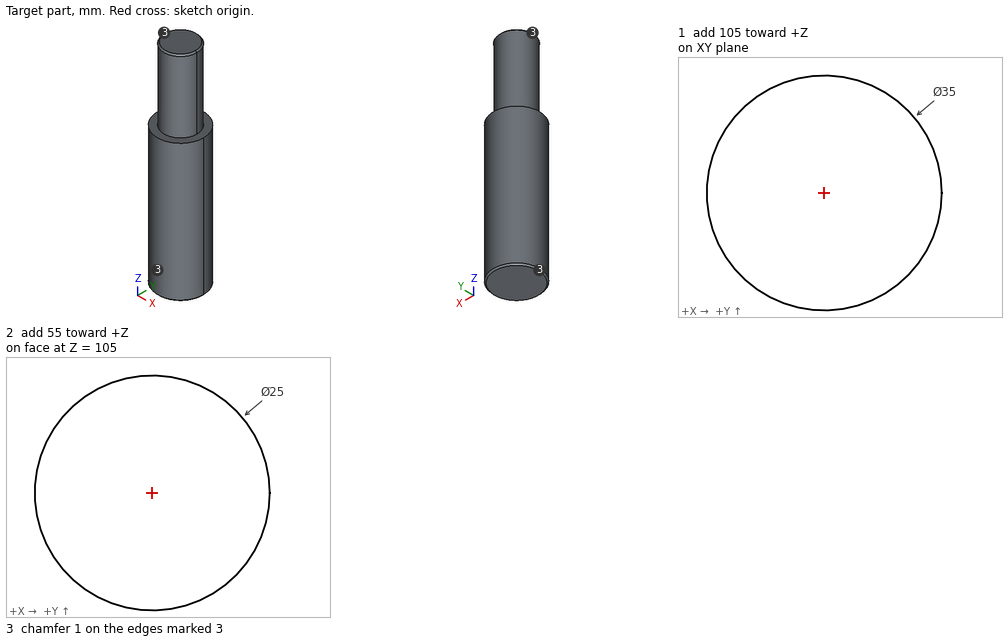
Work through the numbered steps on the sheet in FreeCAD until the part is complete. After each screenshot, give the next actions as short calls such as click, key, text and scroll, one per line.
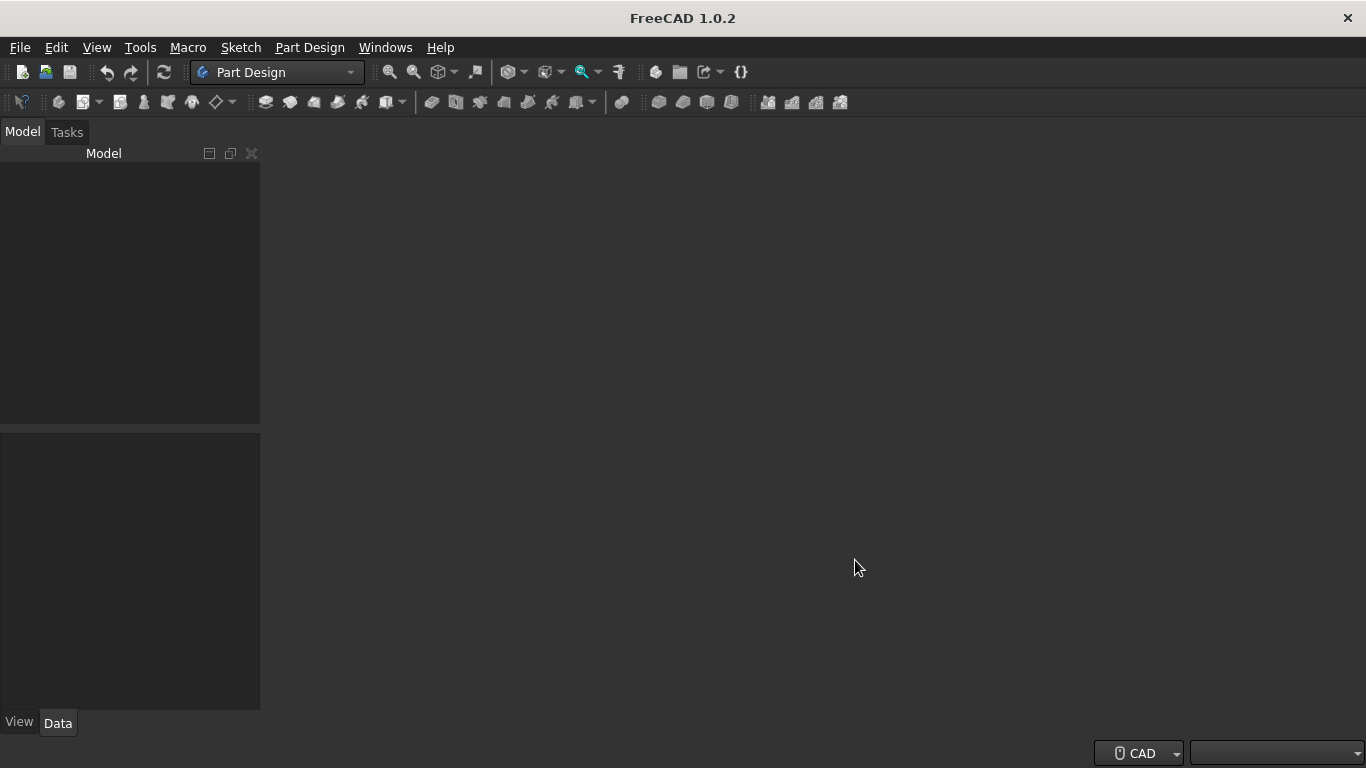
click(22, 72)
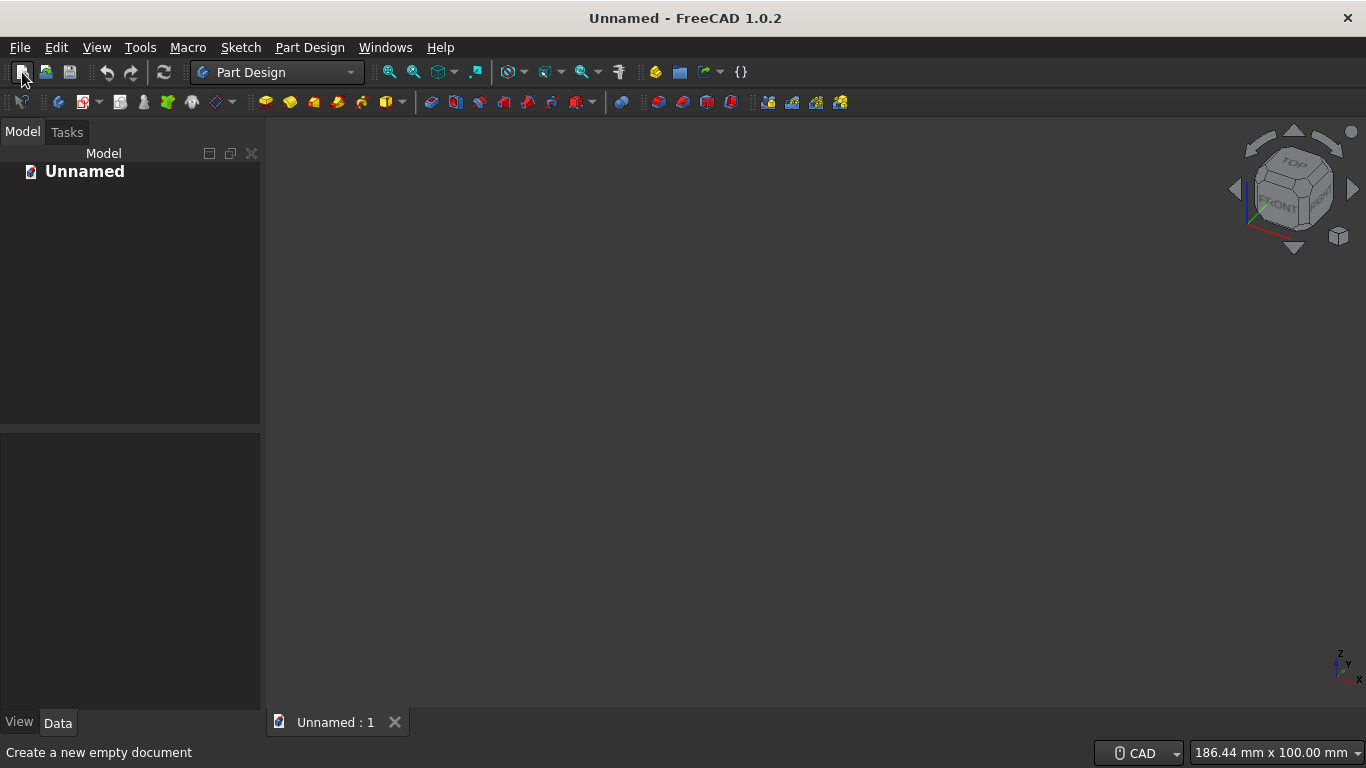
click(84, 102)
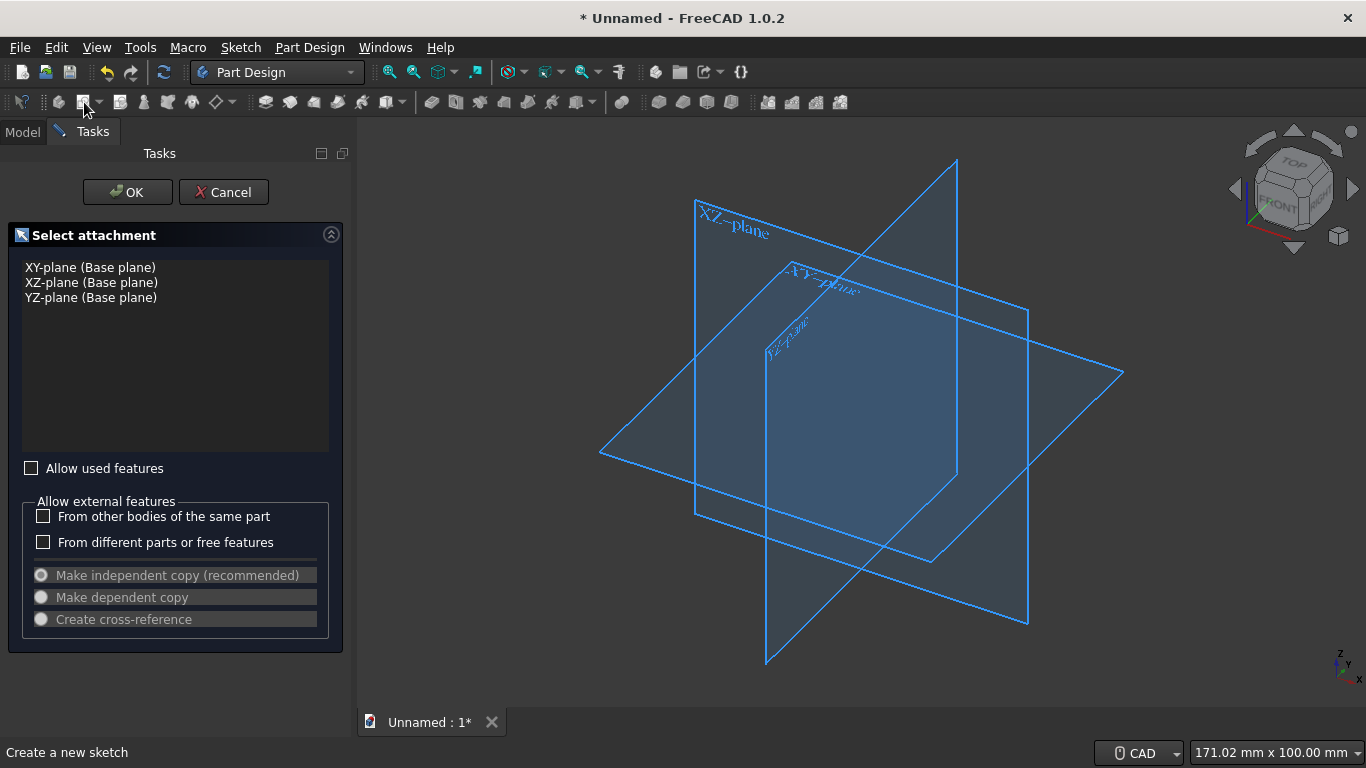
click(82, 268)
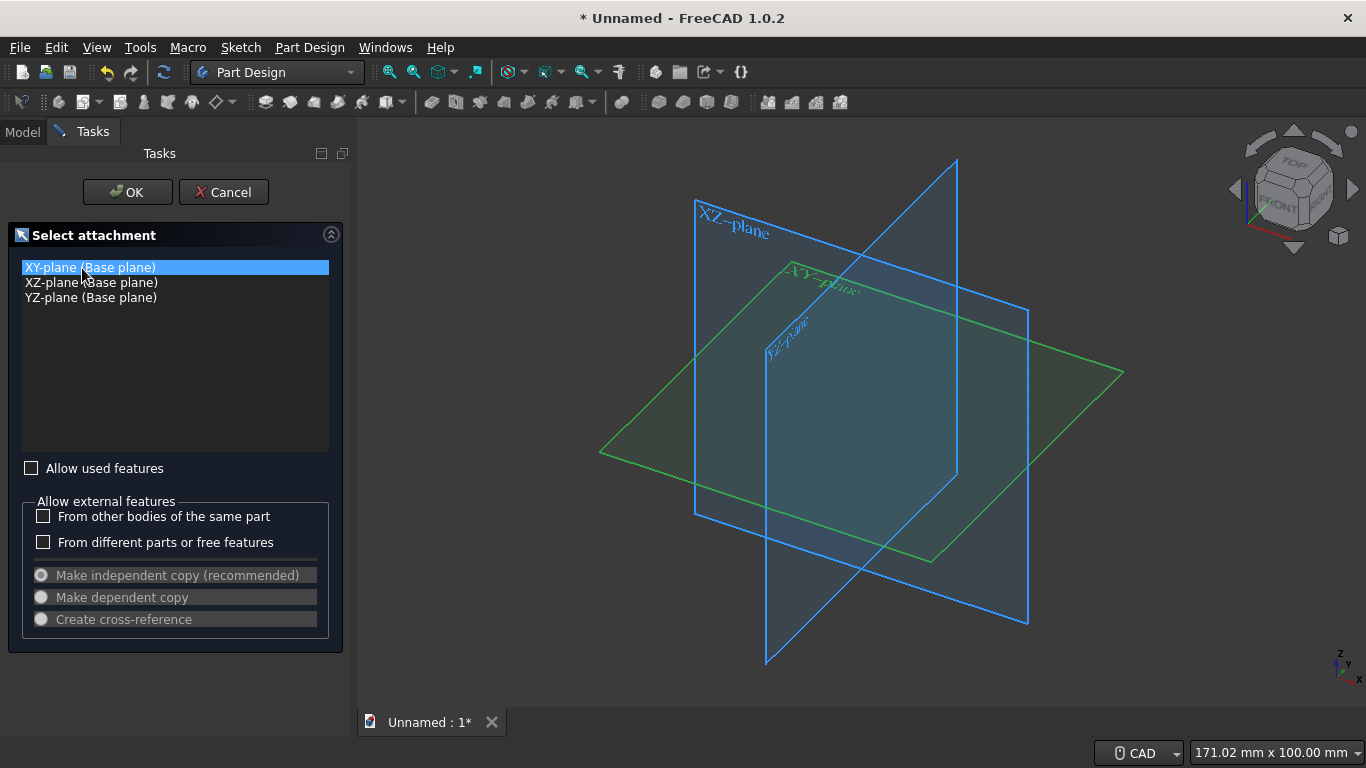
click(128, 192)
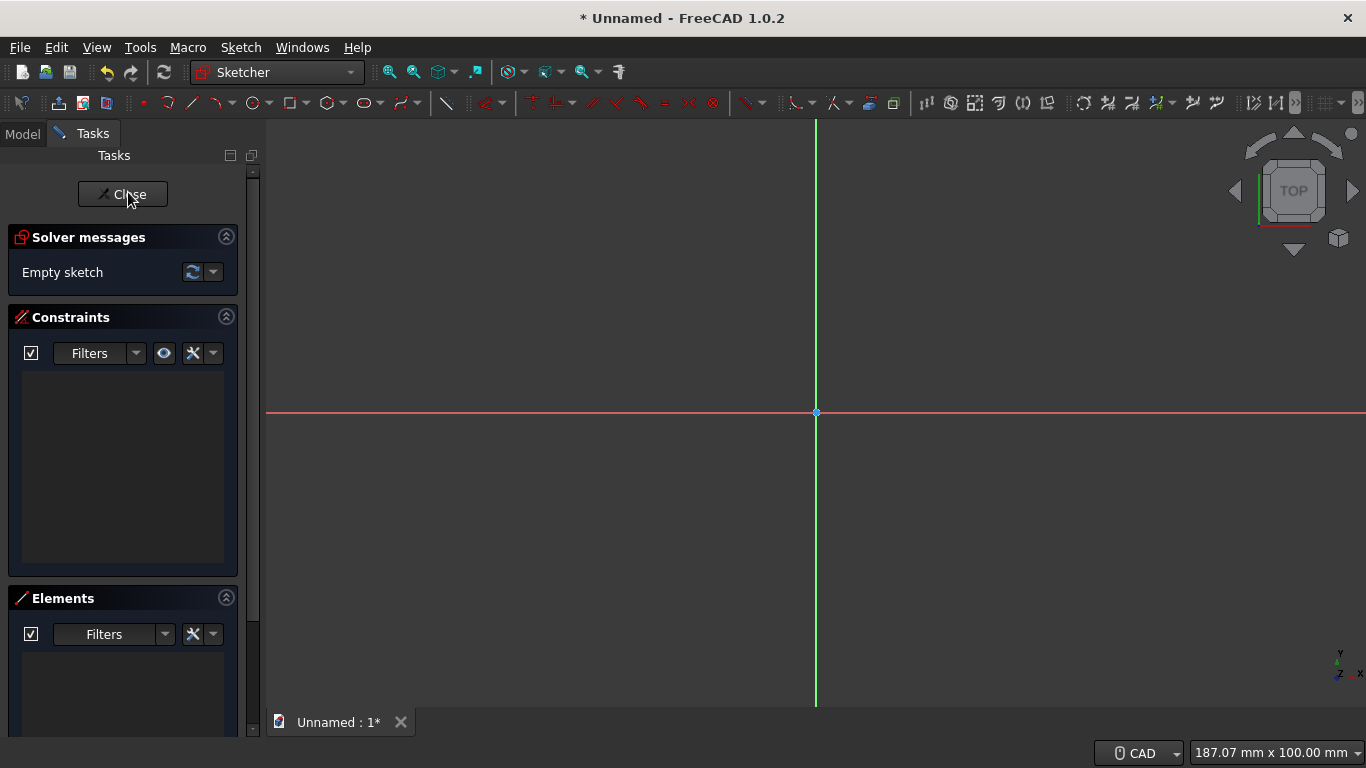
scroll(899, 413, up, 3)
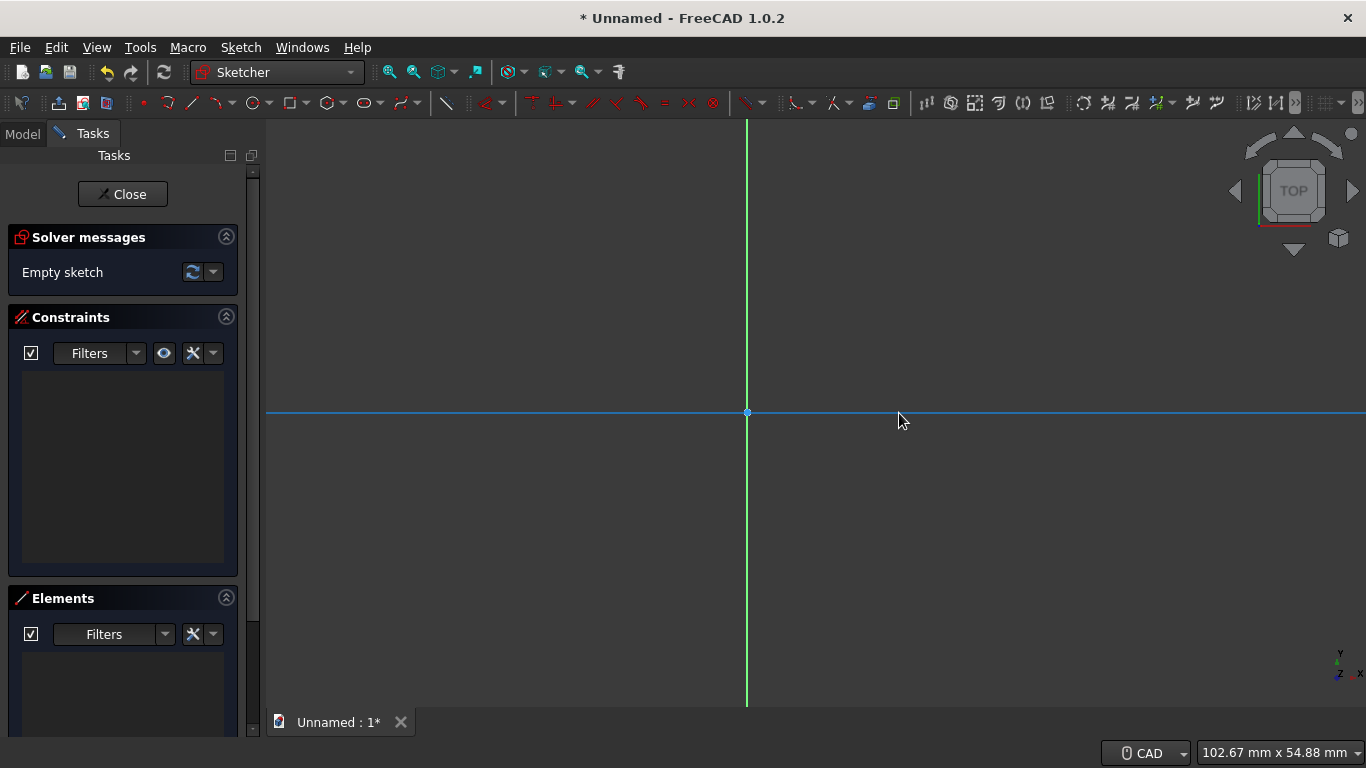
click(254, 104)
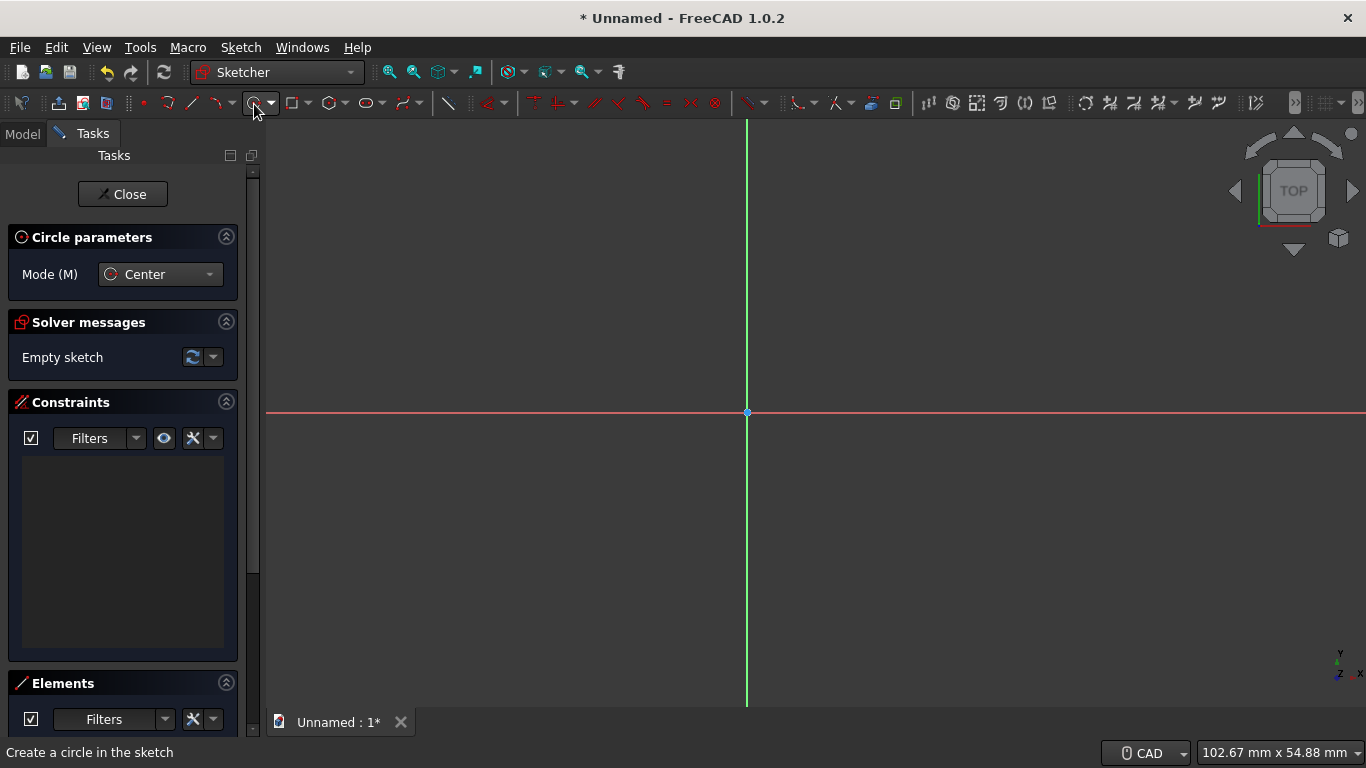
click(747, 413)
click(880, 280)
key(Escape)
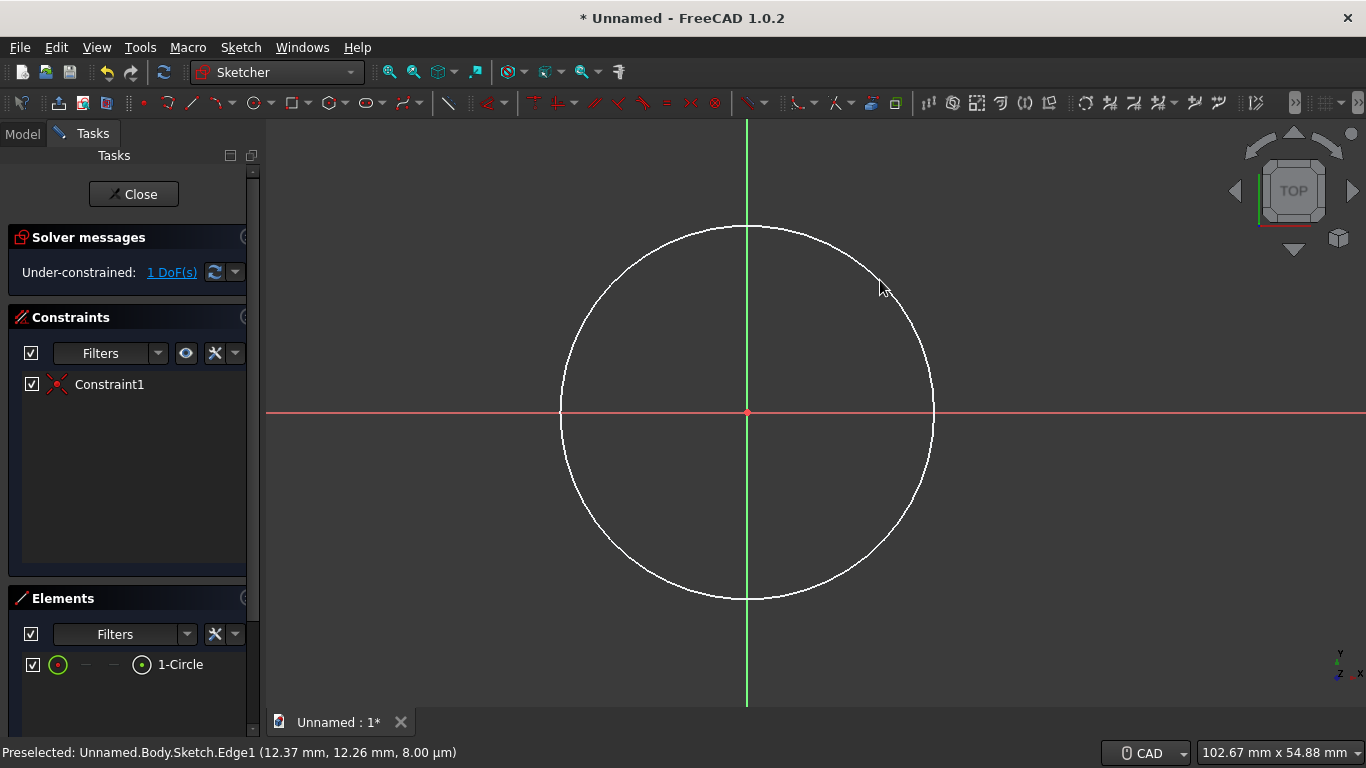
click(488, 104)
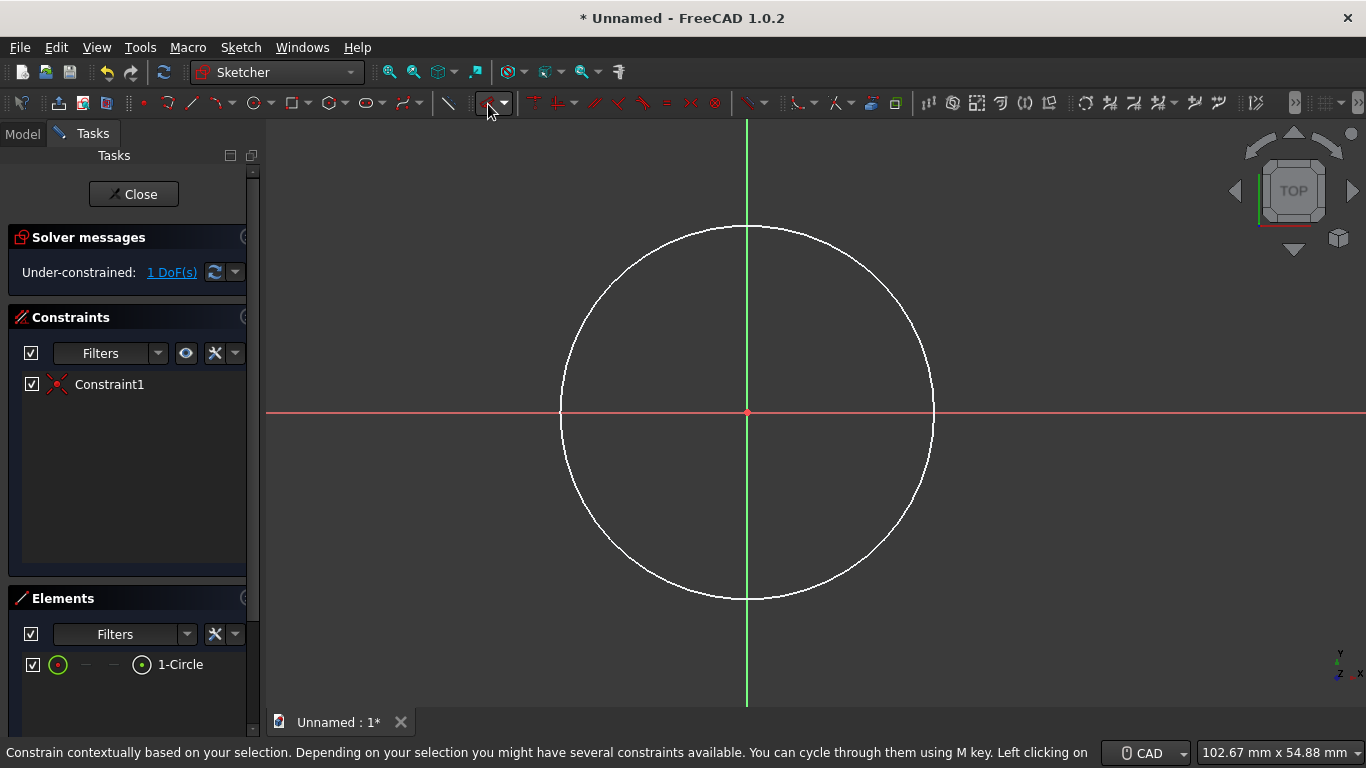
click(879, 280)
click(902, 257)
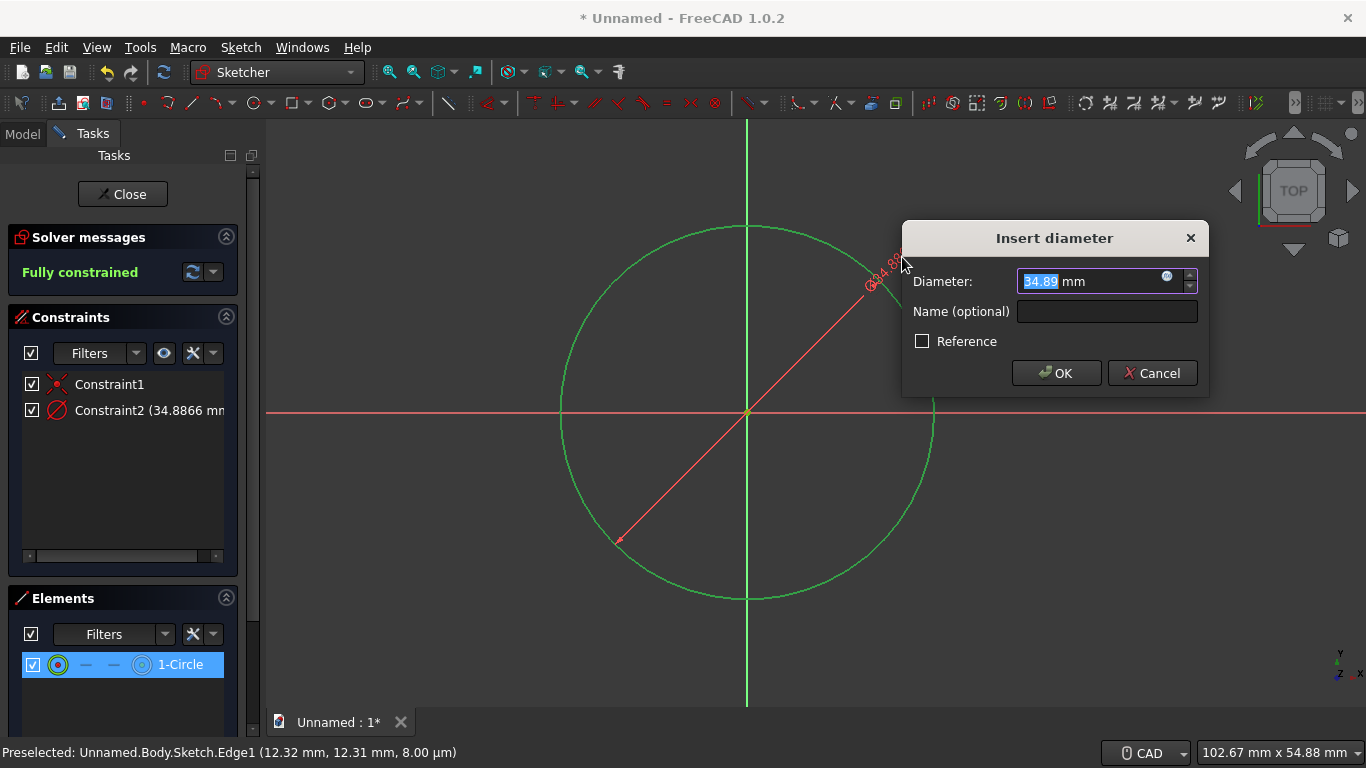
text(35)
key(Return)
key(Escape)